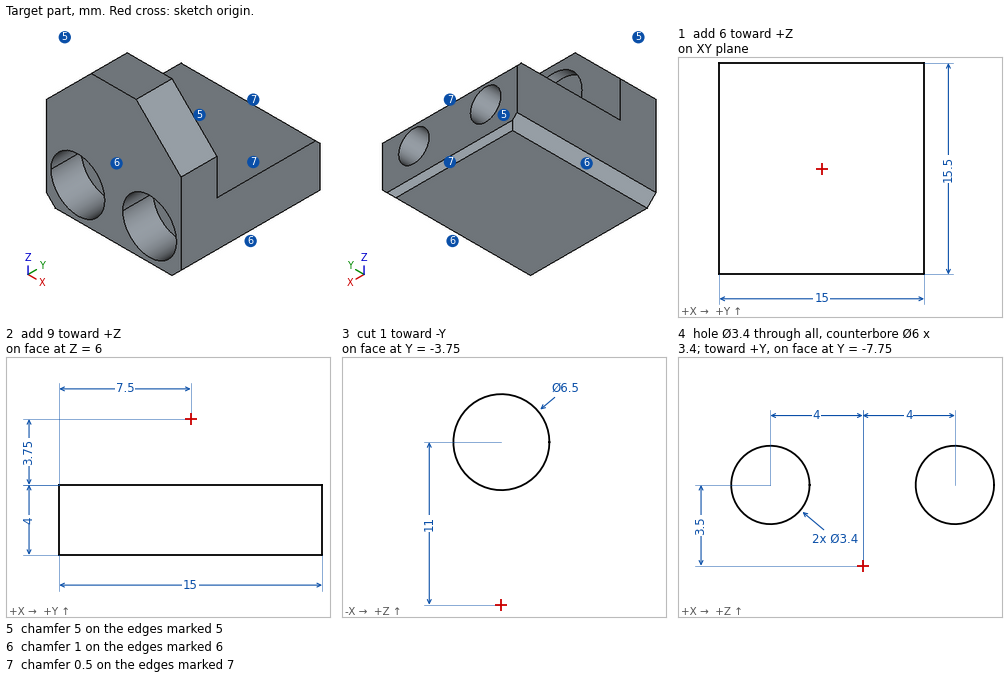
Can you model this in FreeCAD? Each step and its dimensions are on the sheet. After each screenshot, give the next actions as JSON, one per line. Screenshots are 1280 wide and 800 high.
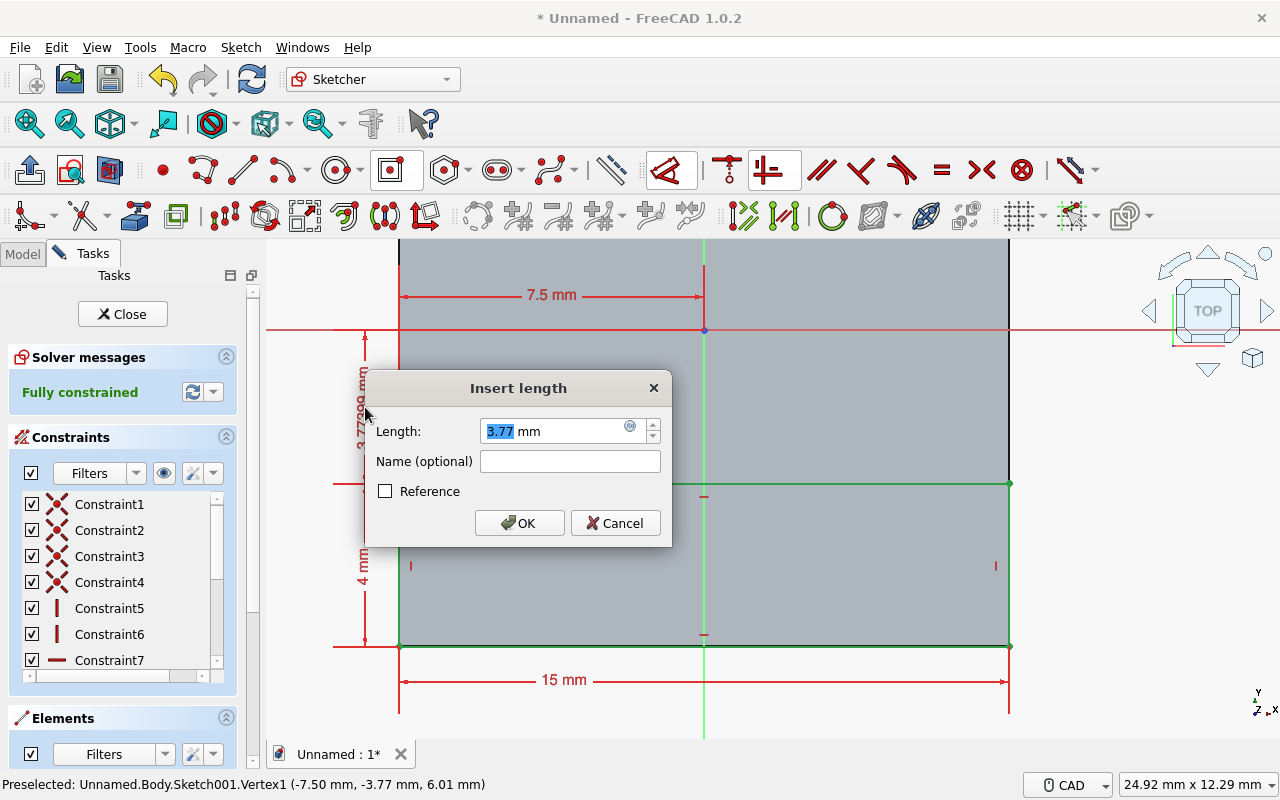
{"action": "type", "text": "3.75"}
{"action": "key", "text": "Return"}
{"action": "key", "text": "Escape"}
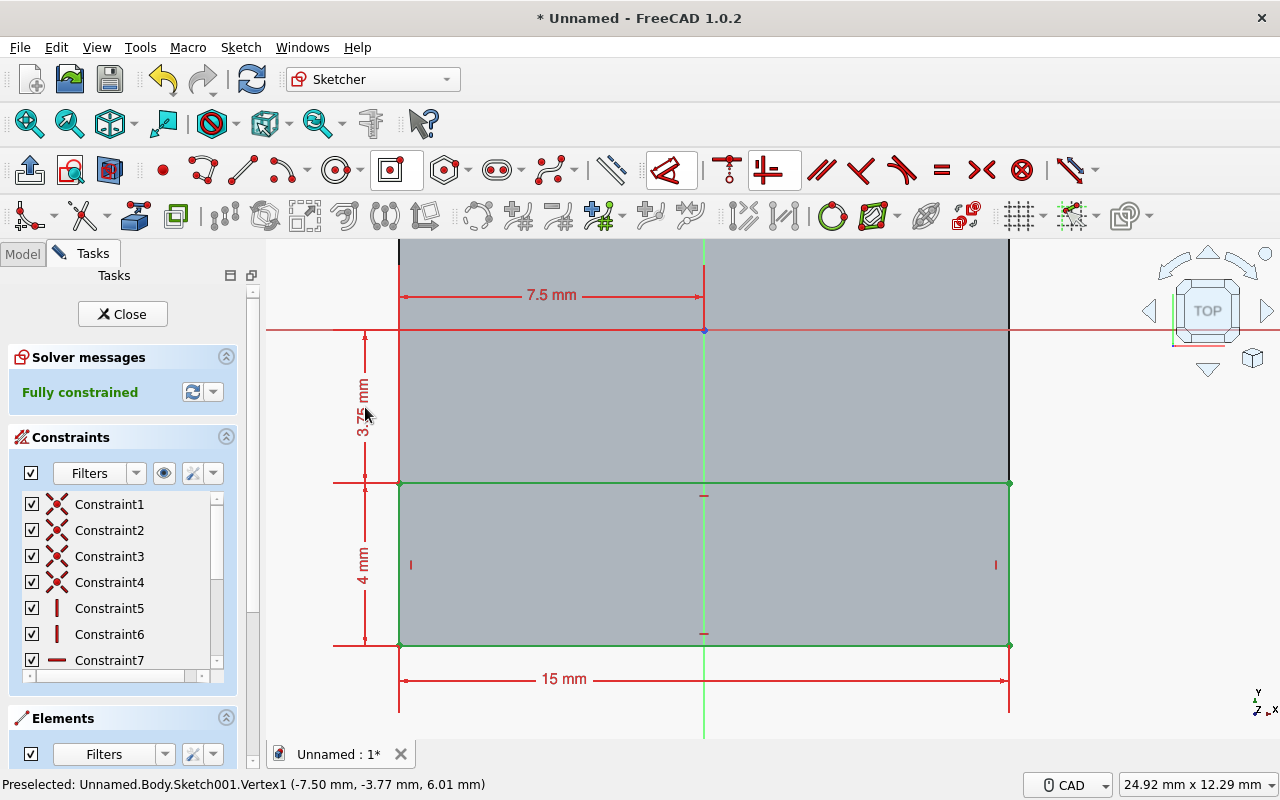
{"action": "left_click", "coordinate": [123, 314]}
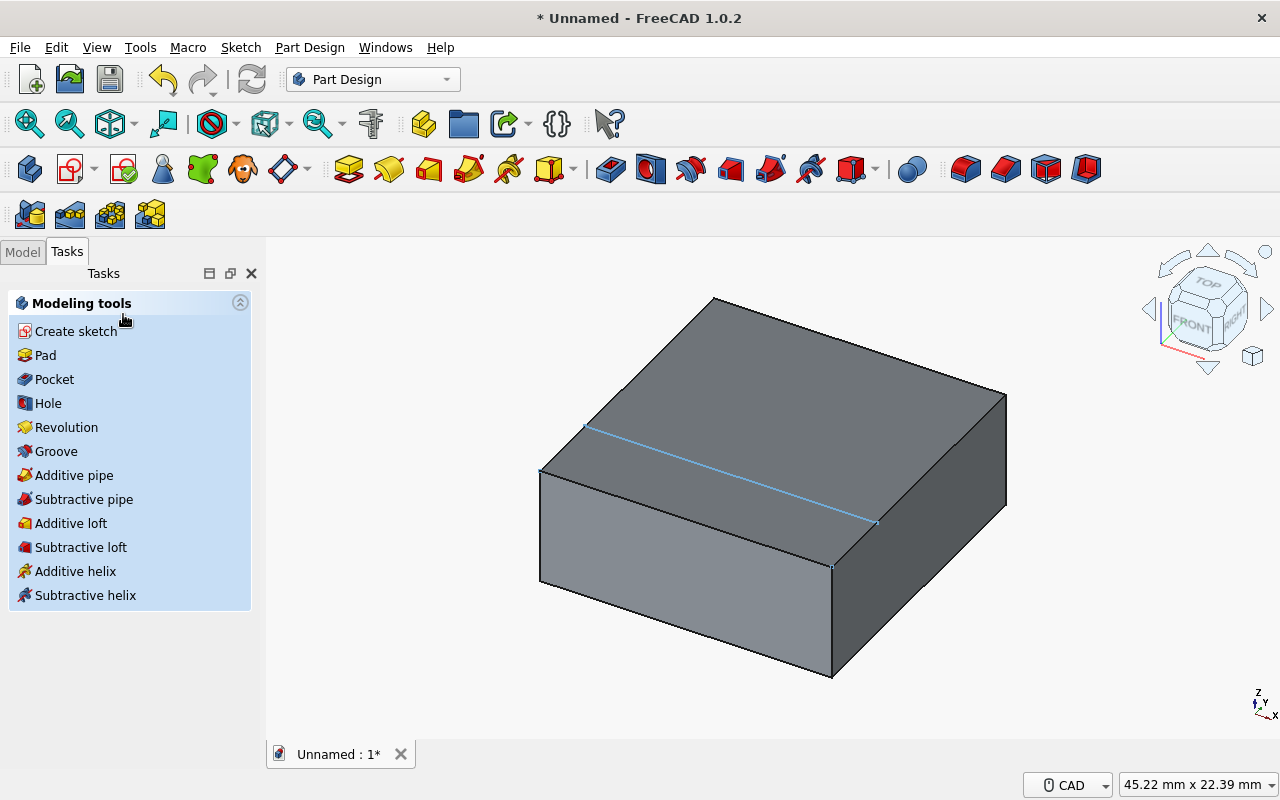
{"action": "left_click", "coordinate": [350, 170]}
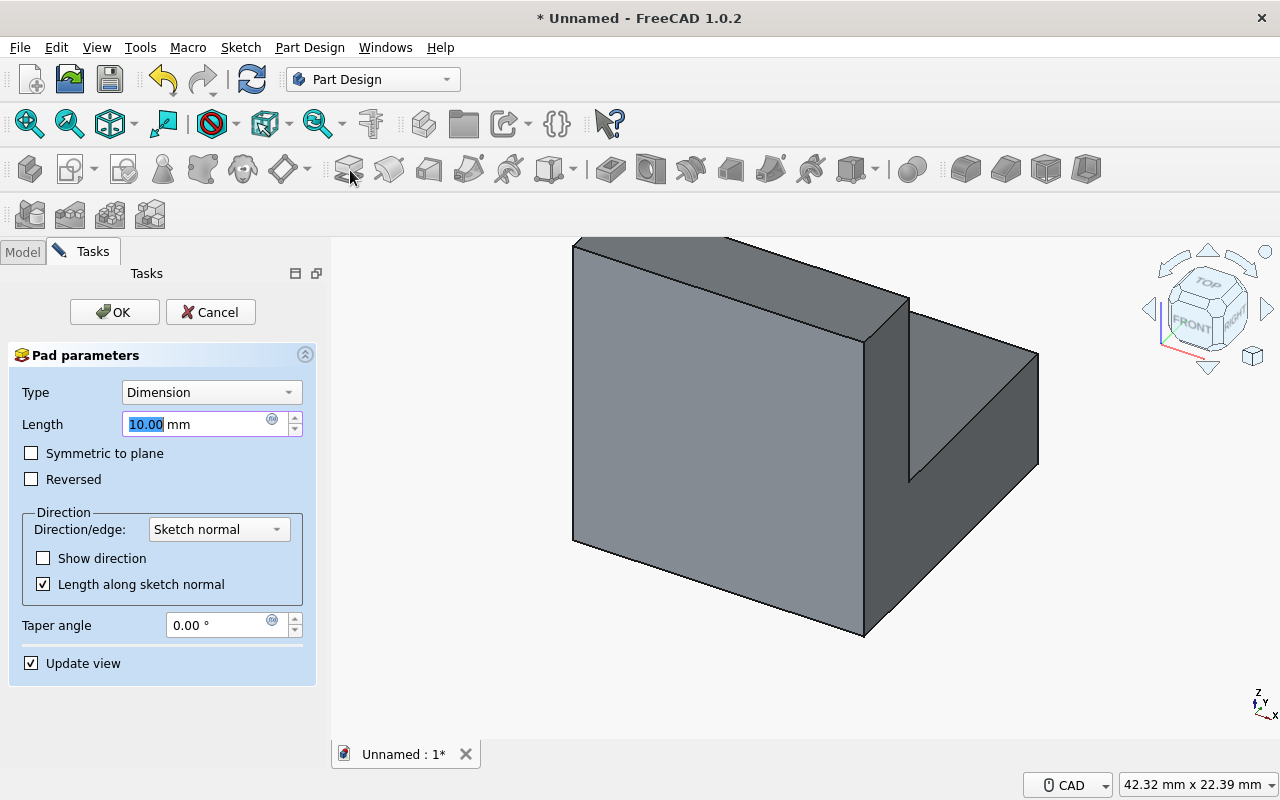
{"action": "type", "text": "9"}
{"action": "key", "text": "Tab"}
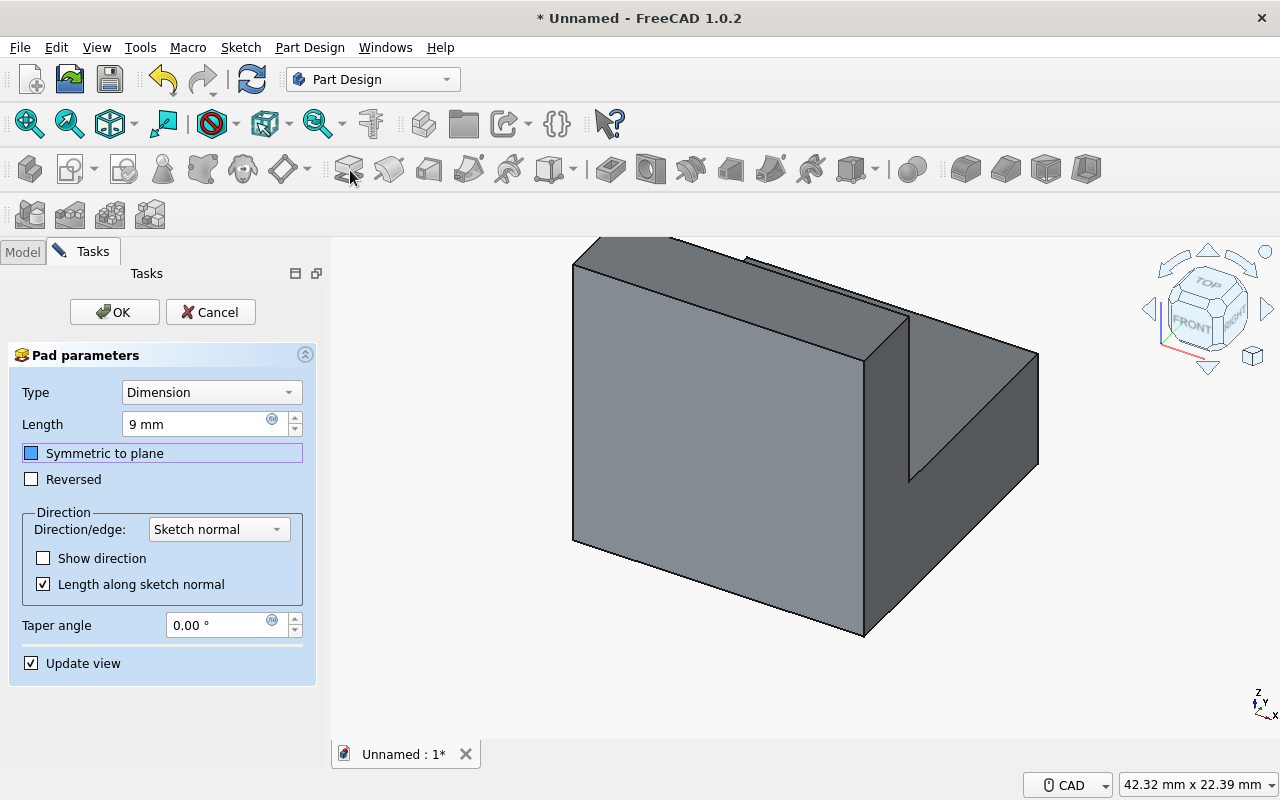
{"action": "left_click", "coordinate": [115, 312]}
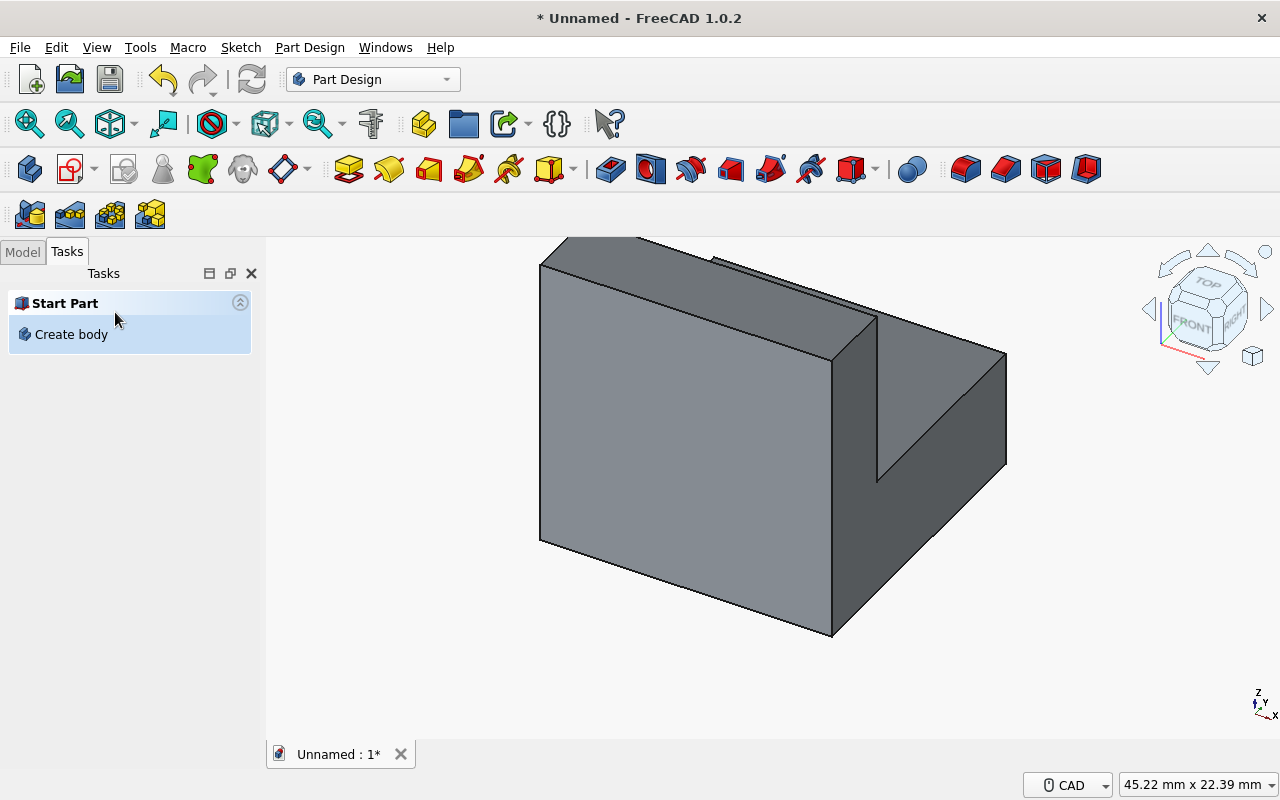
{"action": "key", "text": "v f"}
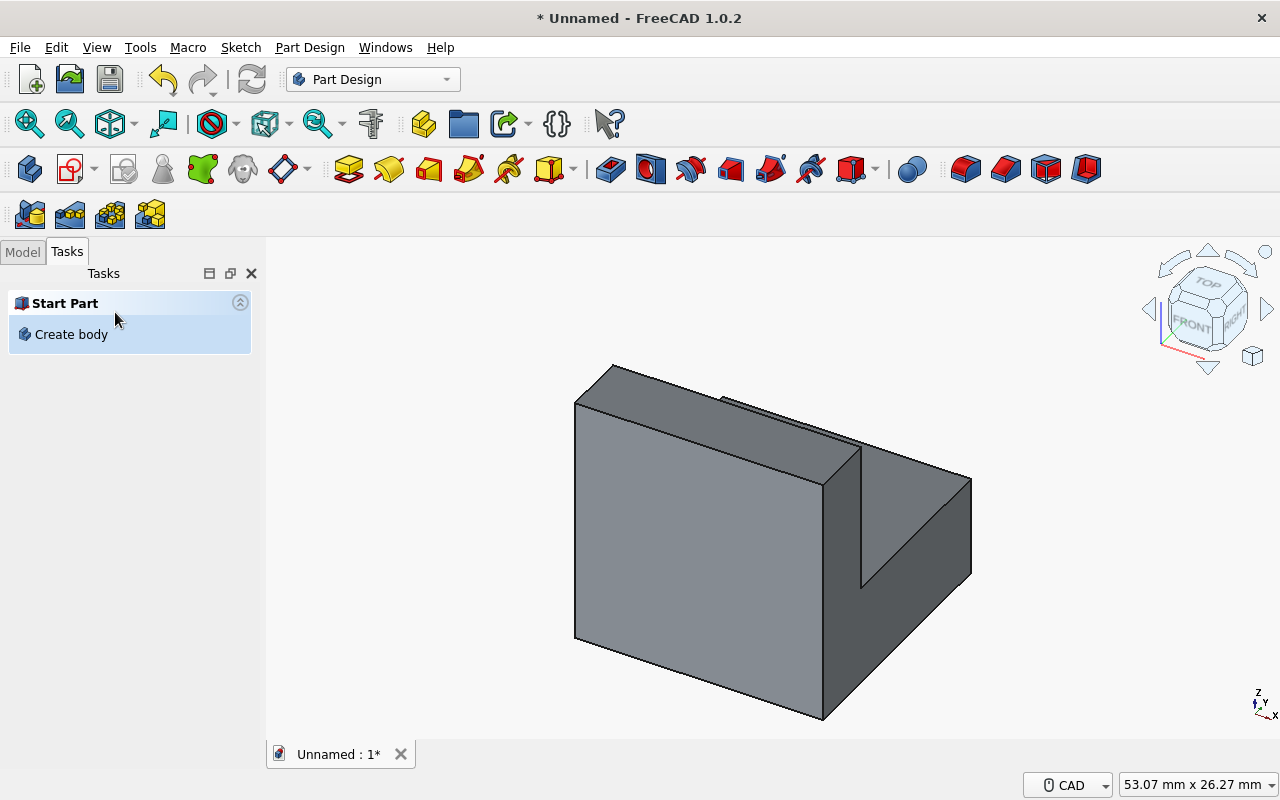
{"action": "key", "text": "4"}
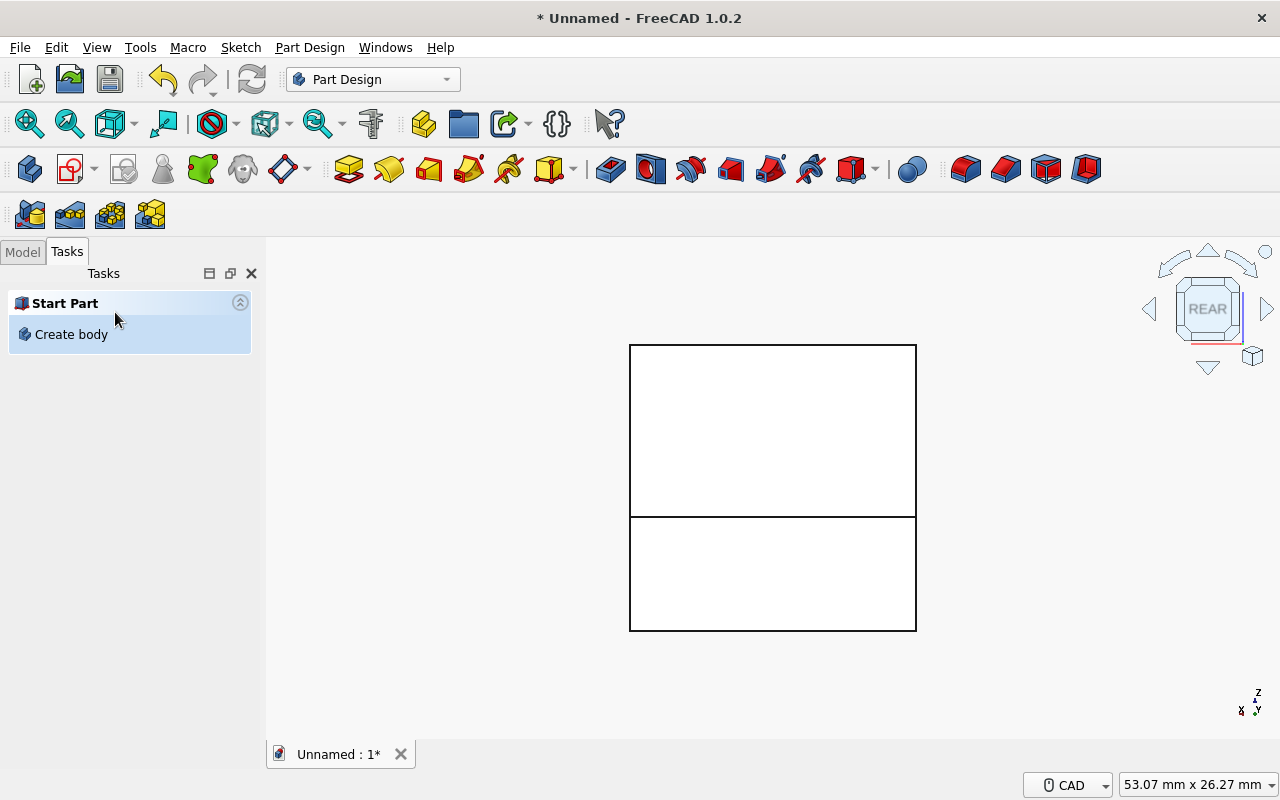
{"action": "left_click", "coordinate": [732, 430]}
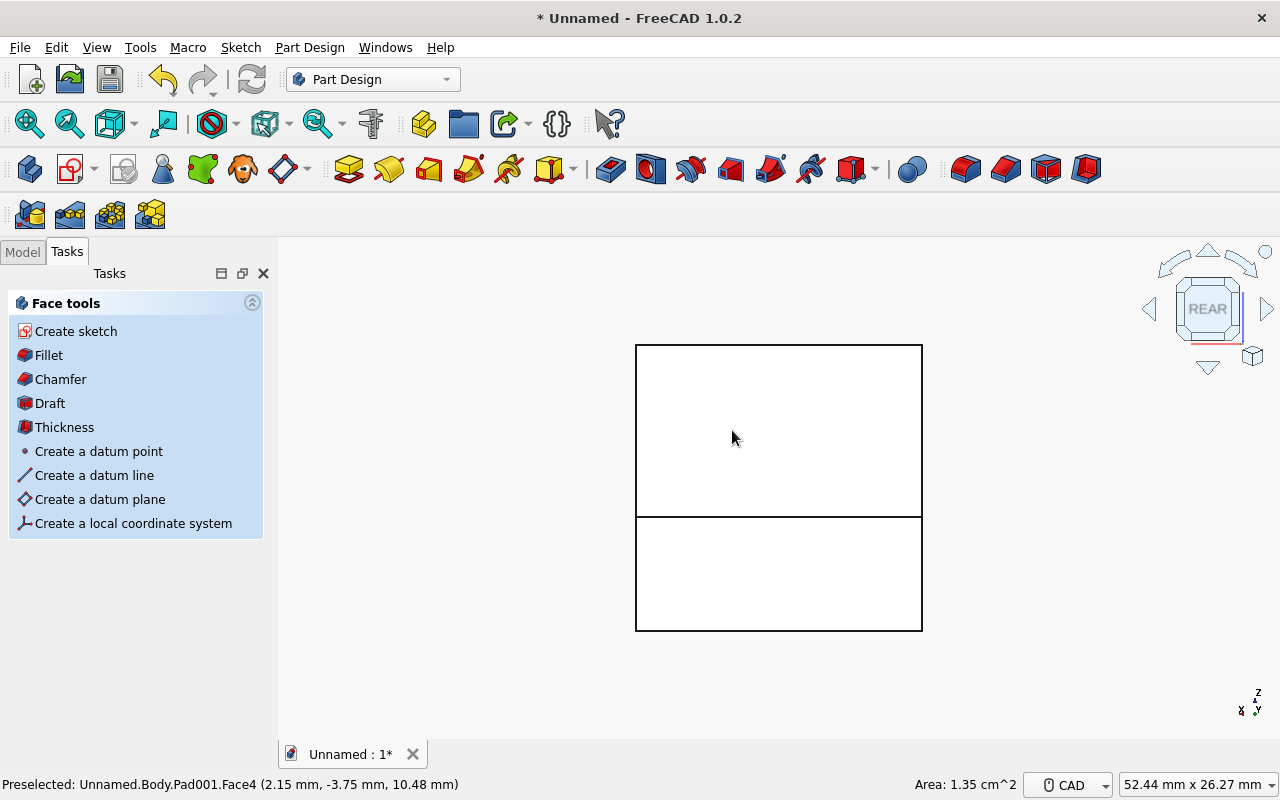
{"action": "left_click", "coordinate": [70, 170]}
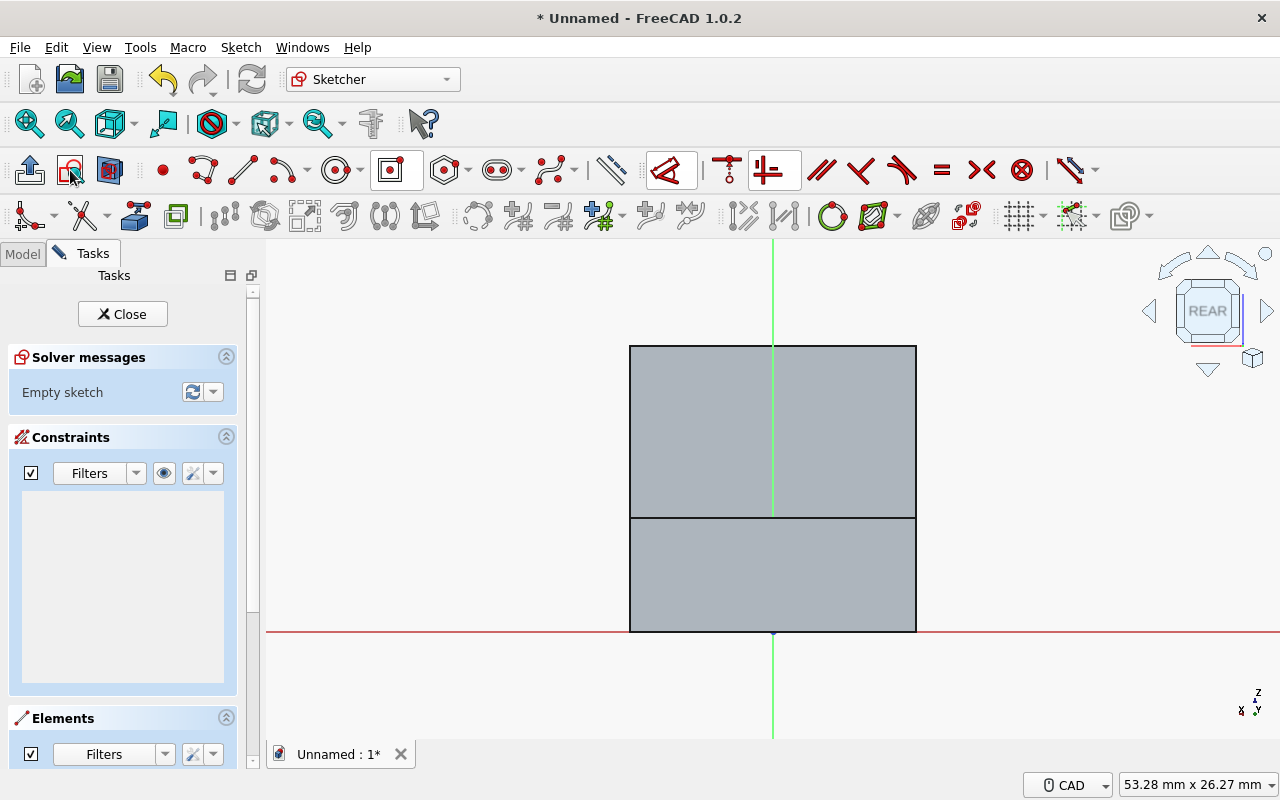
{"action": "key", "text": "g c"}